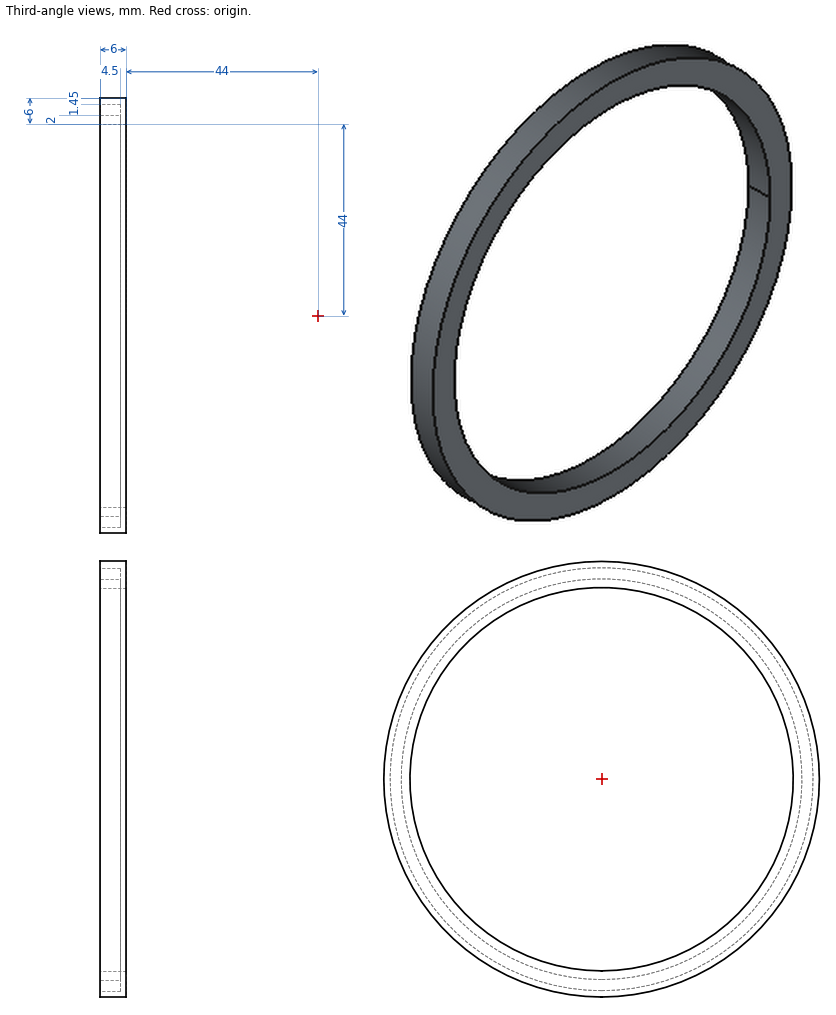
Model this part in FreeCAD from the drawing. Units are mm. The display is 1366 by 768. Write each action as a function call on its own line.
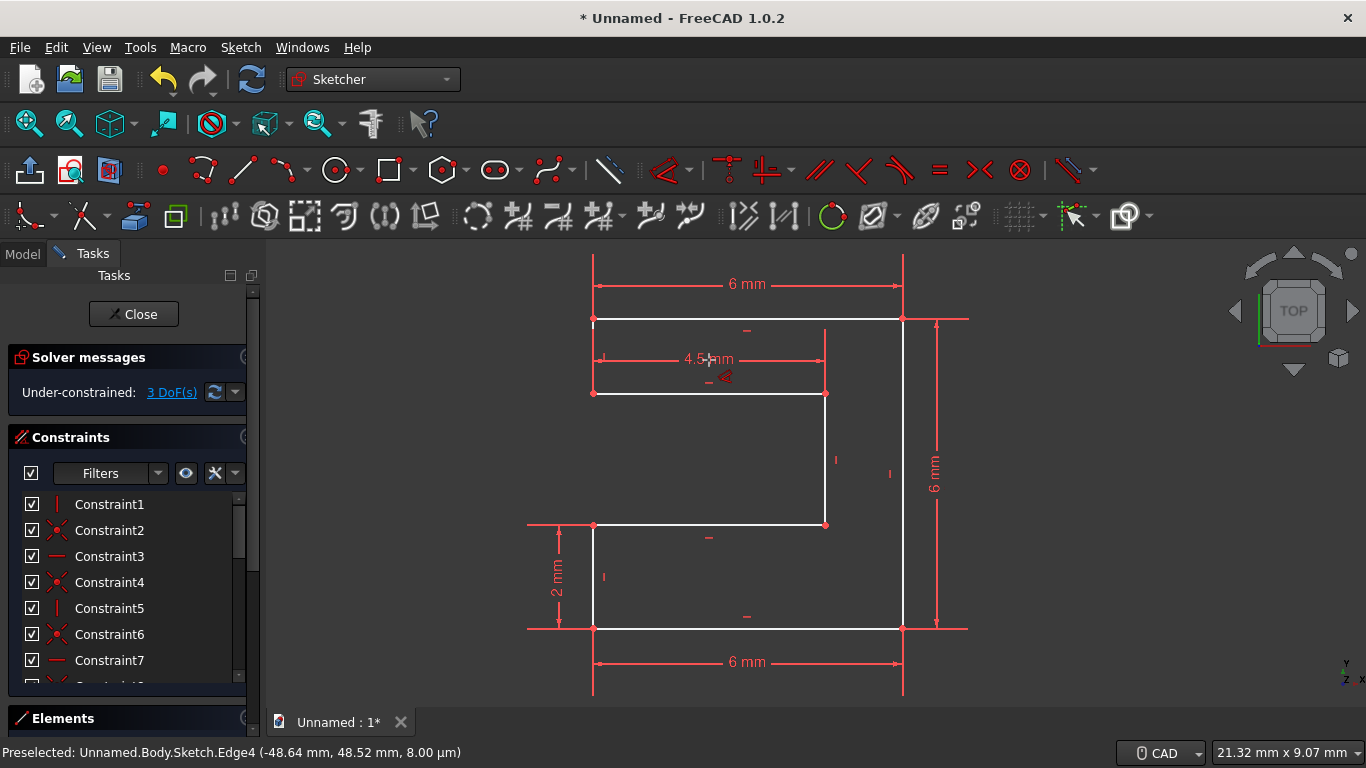
click(903, 629)
click(1052, 595)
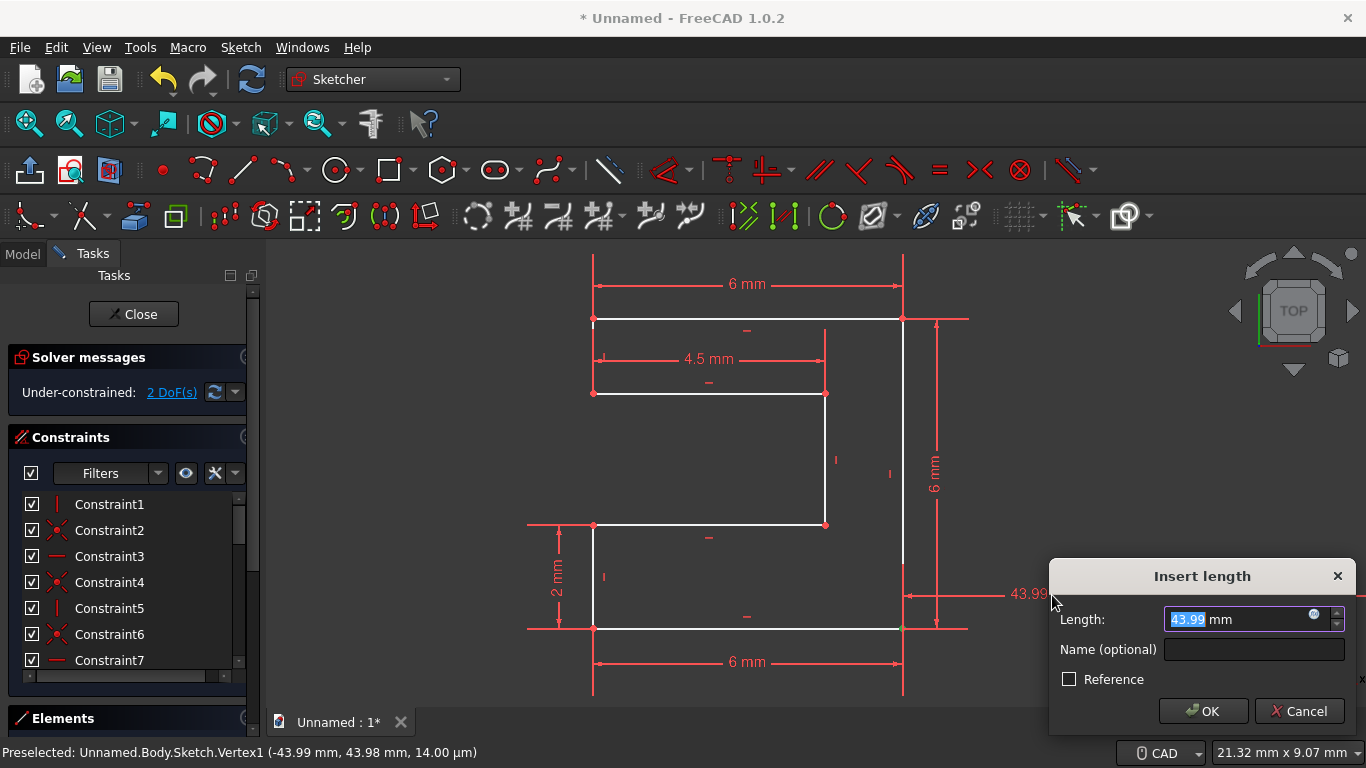
text(44)
key(Return)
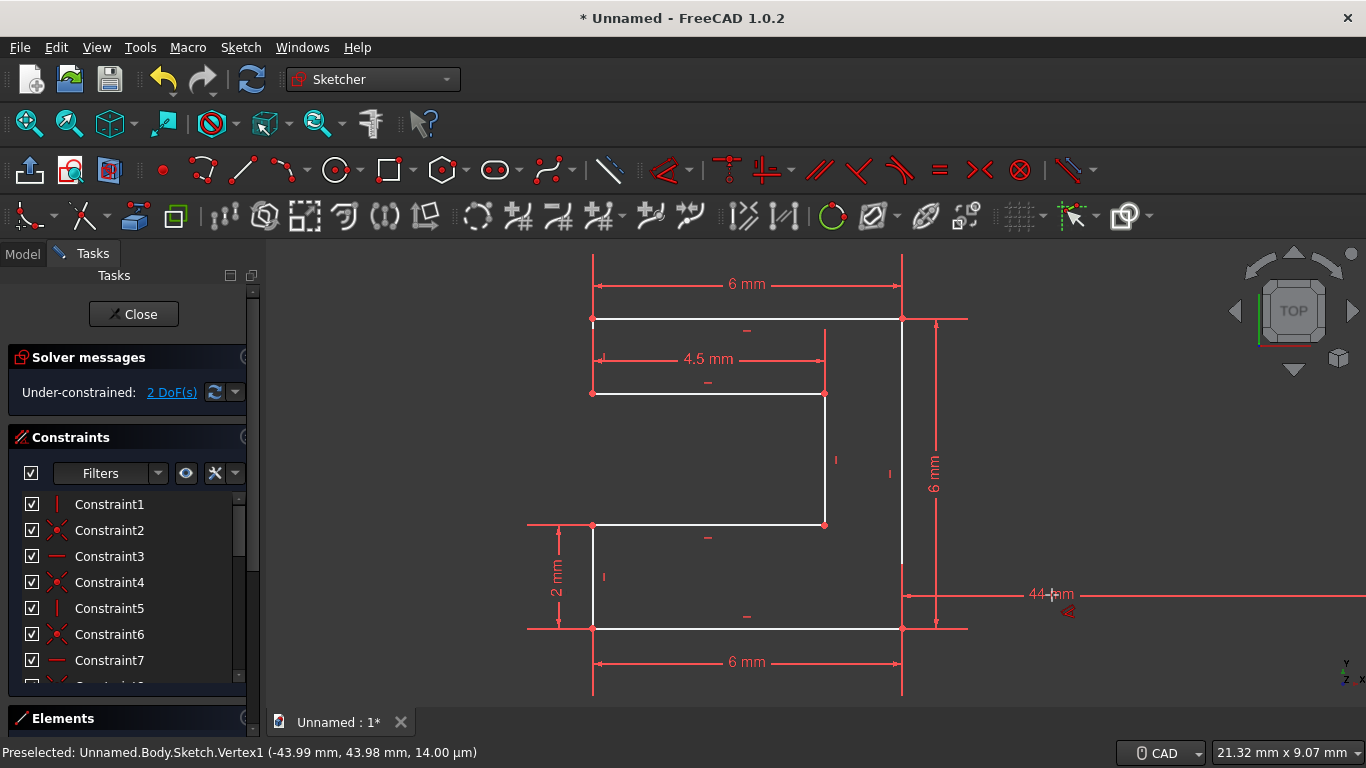
click(902, 629)
click(868, 654)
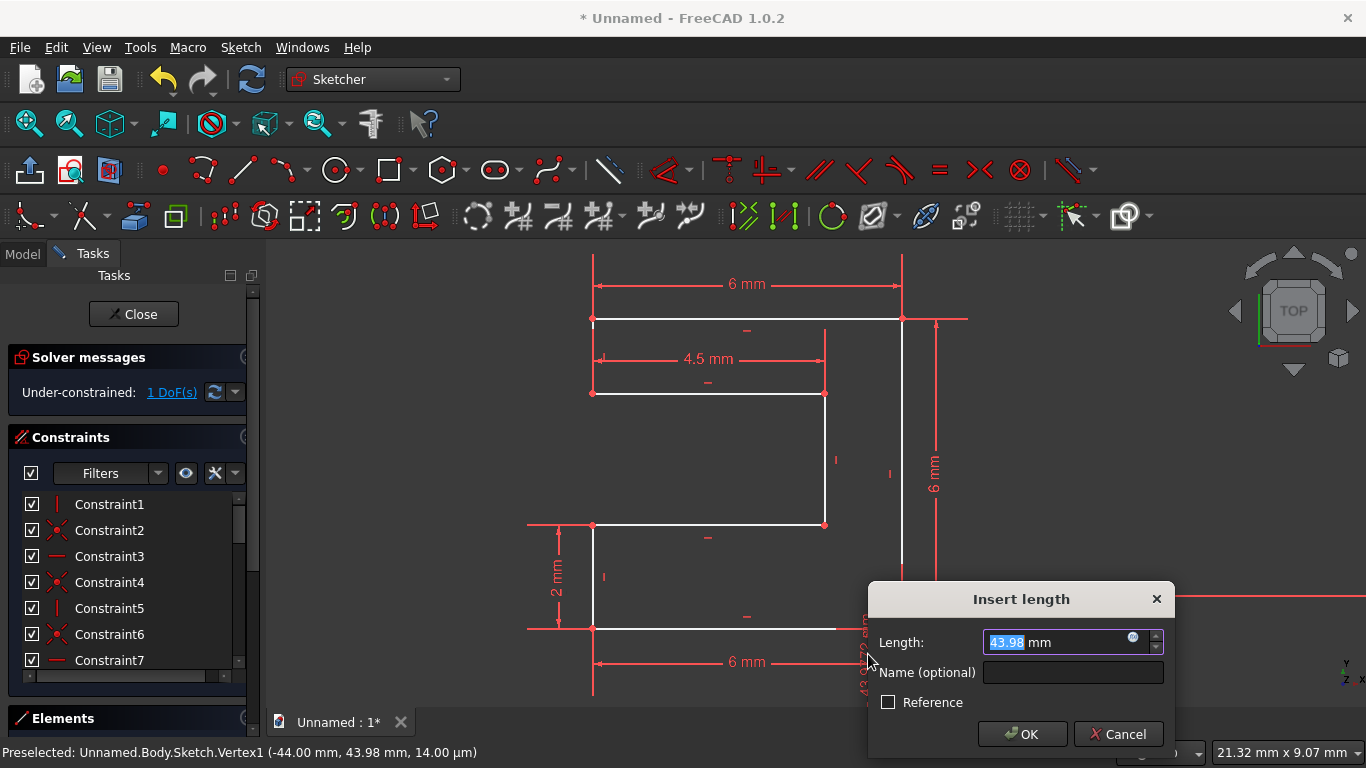
text(44)
key(Return)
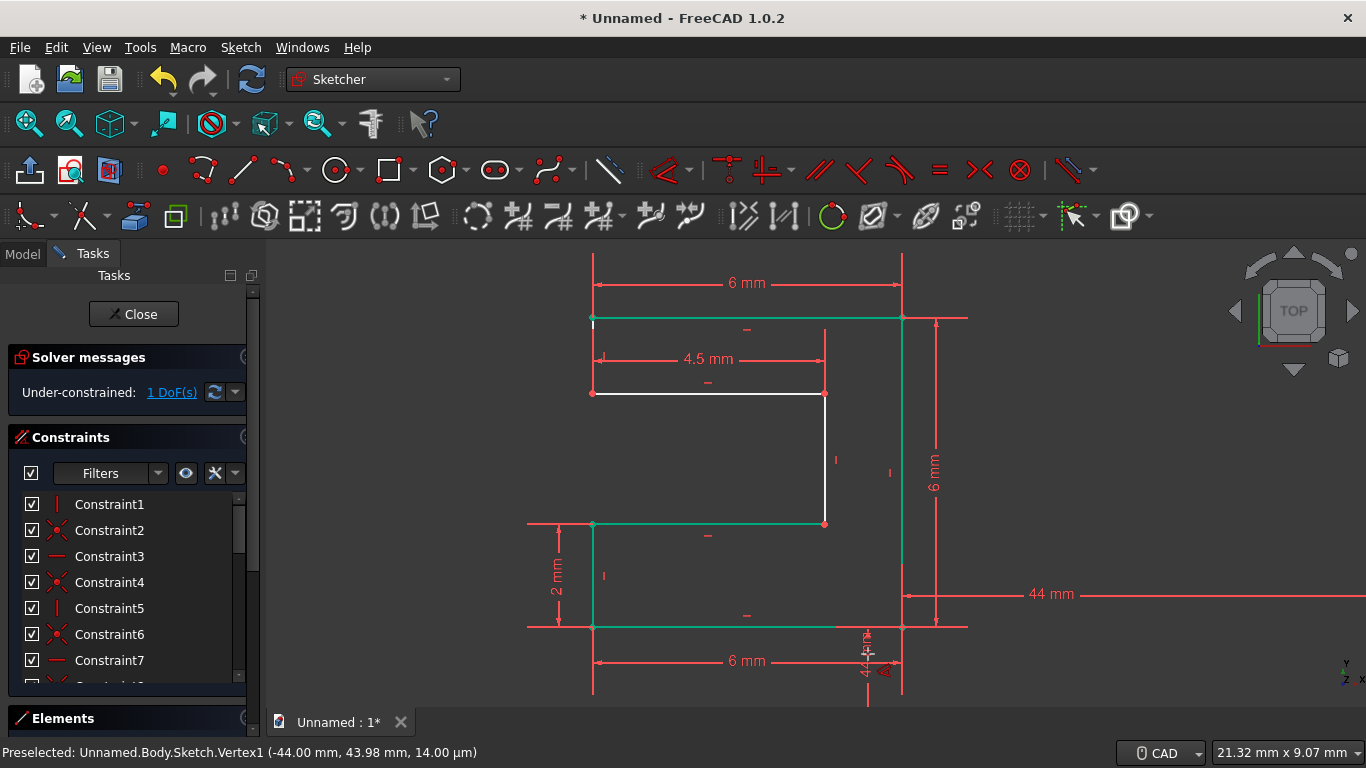
click(593, 341)
click(559, 356)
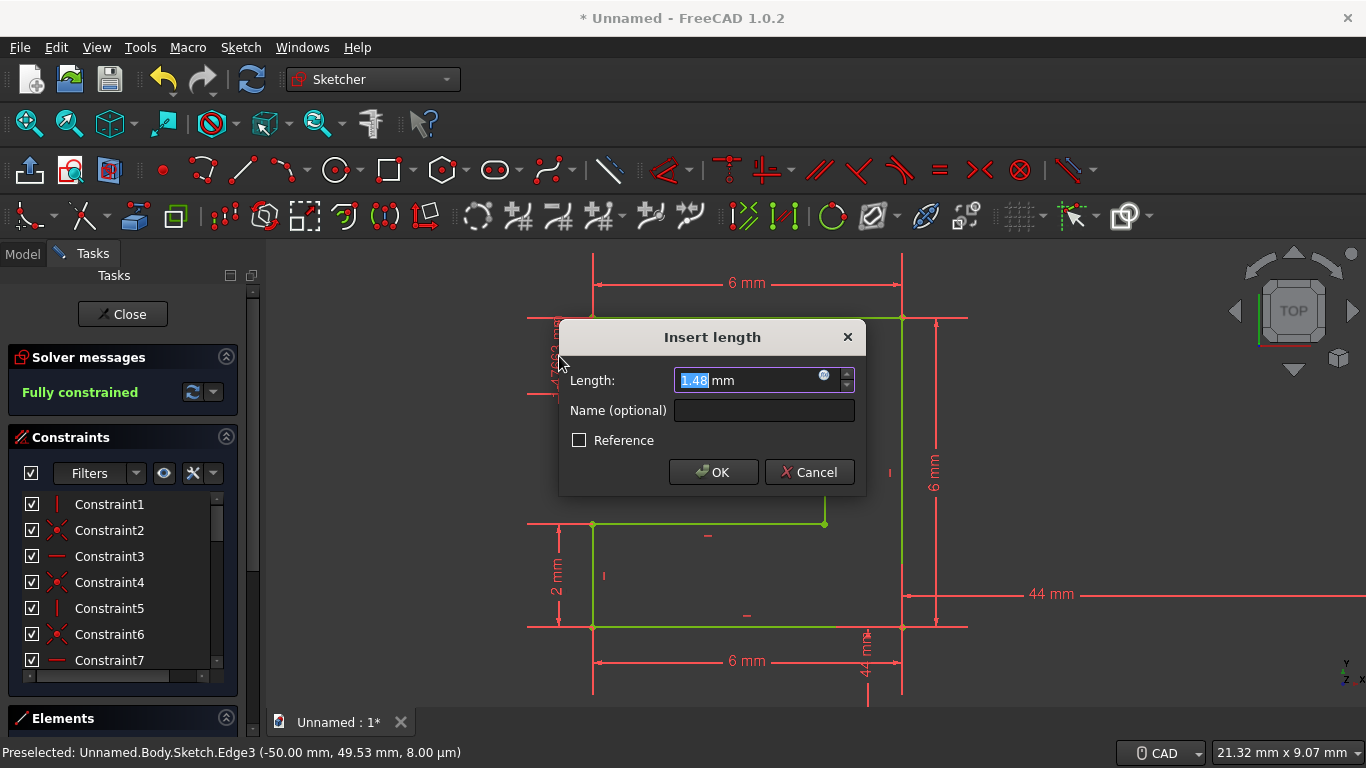
text(1.45)
key(Return)
key(Escape)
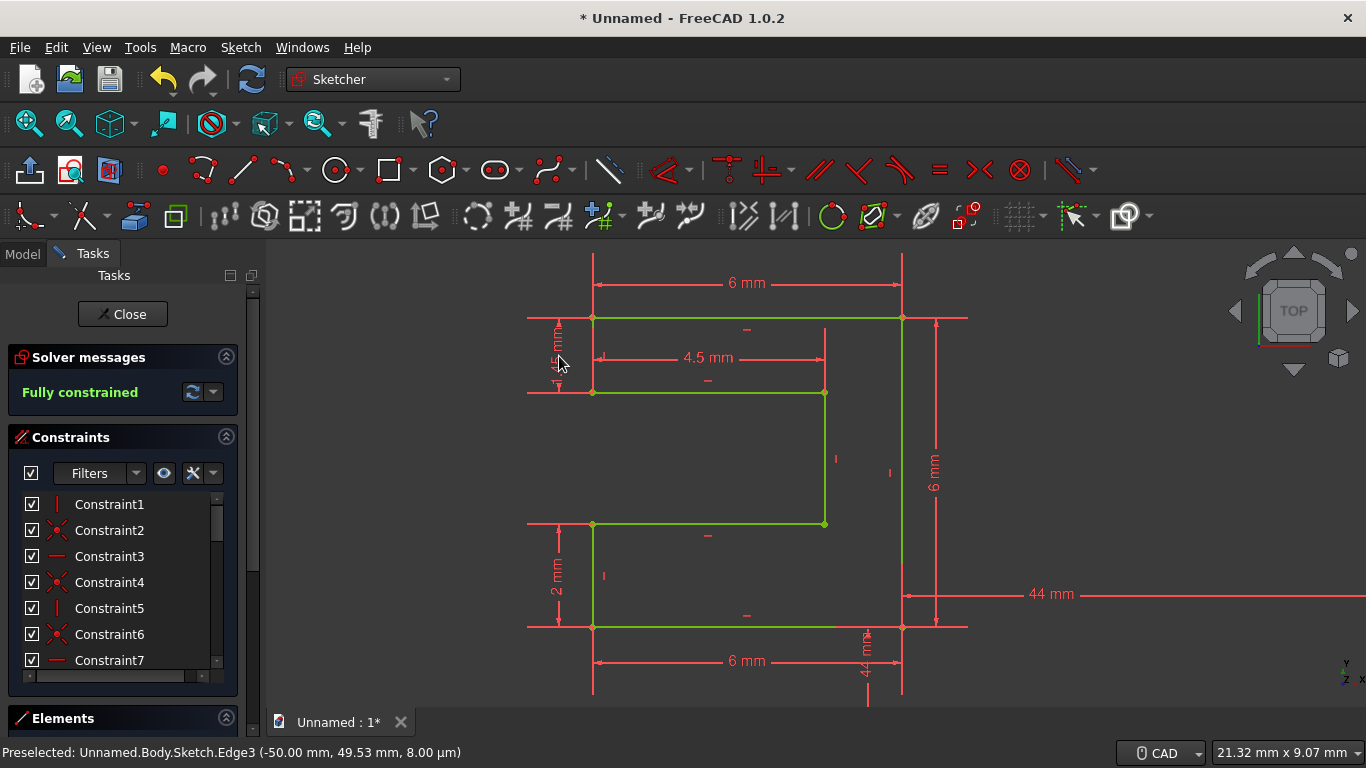
click(123, 314)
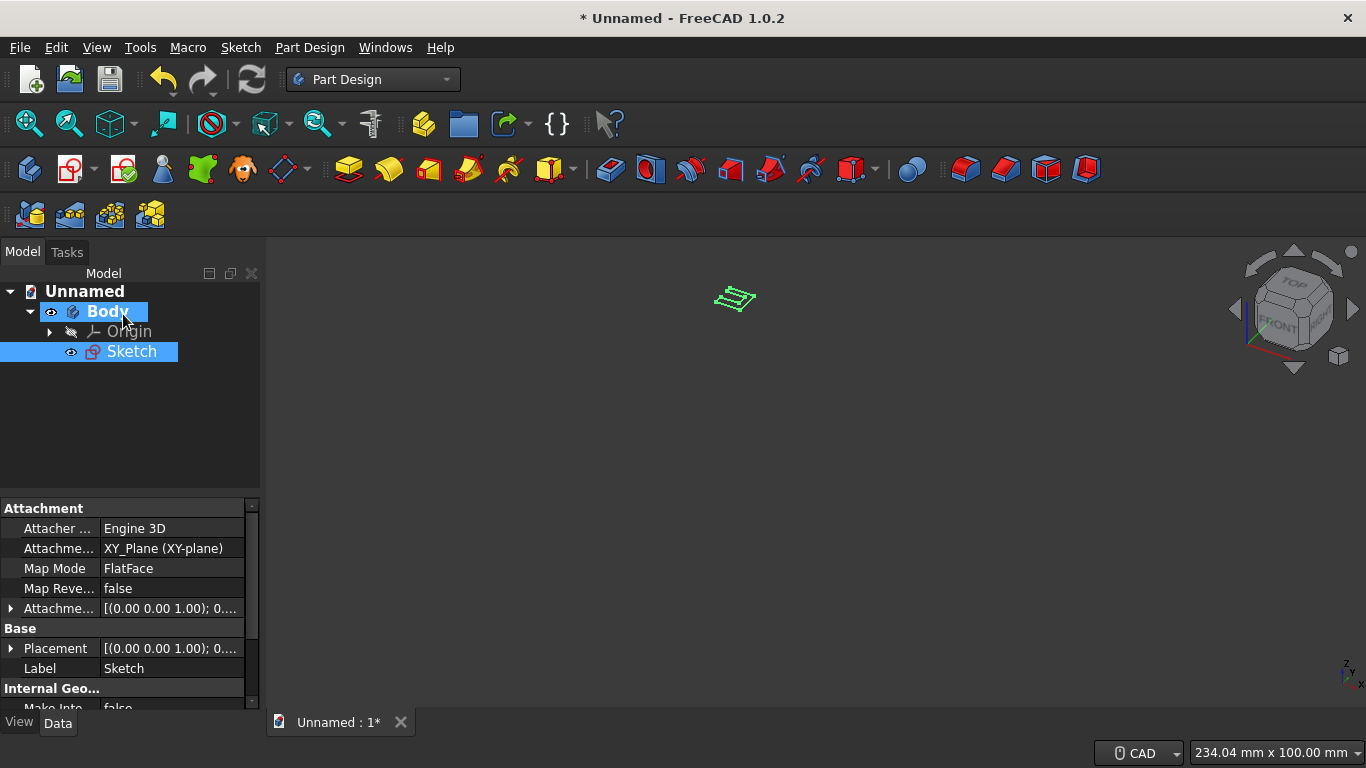
click(390, 170)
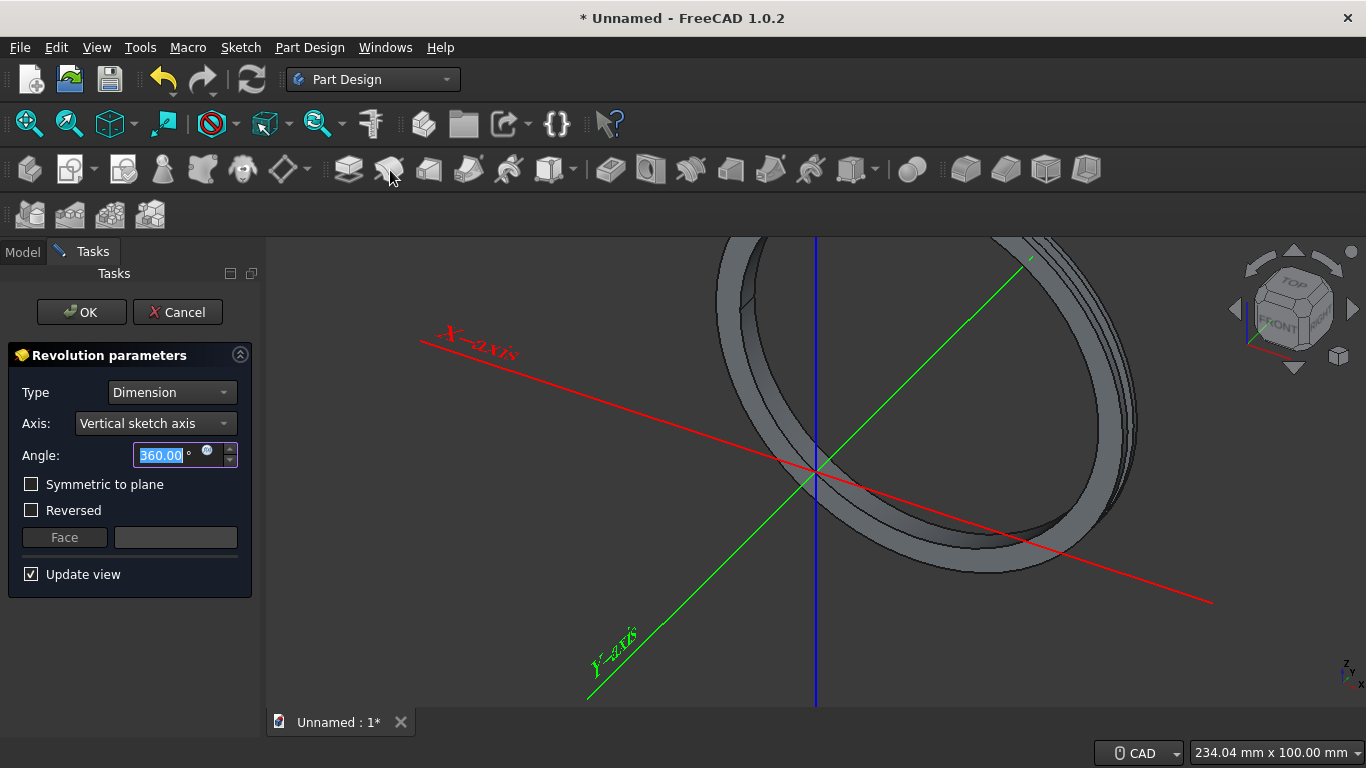
click(156, 424)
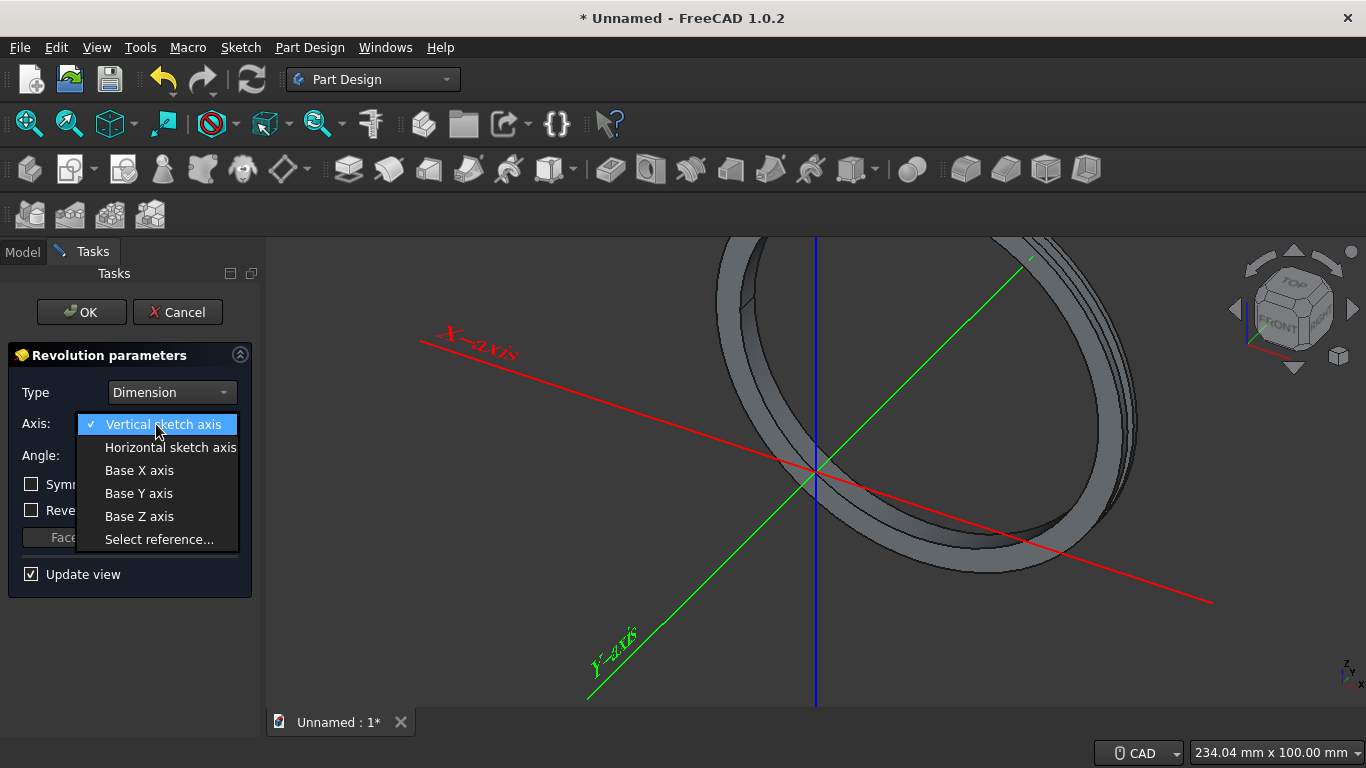
click(156, 448)